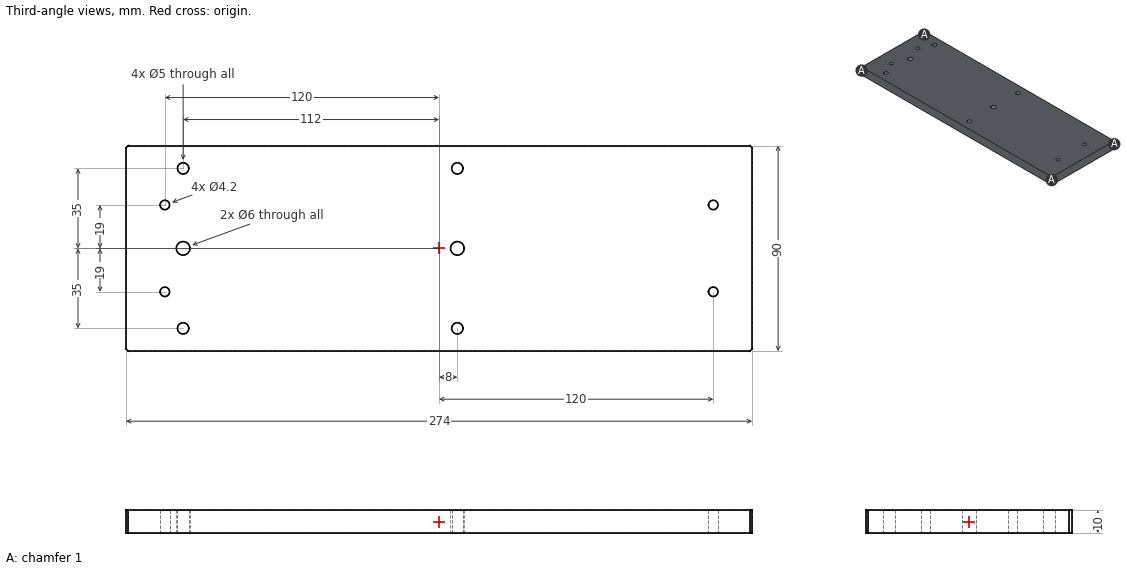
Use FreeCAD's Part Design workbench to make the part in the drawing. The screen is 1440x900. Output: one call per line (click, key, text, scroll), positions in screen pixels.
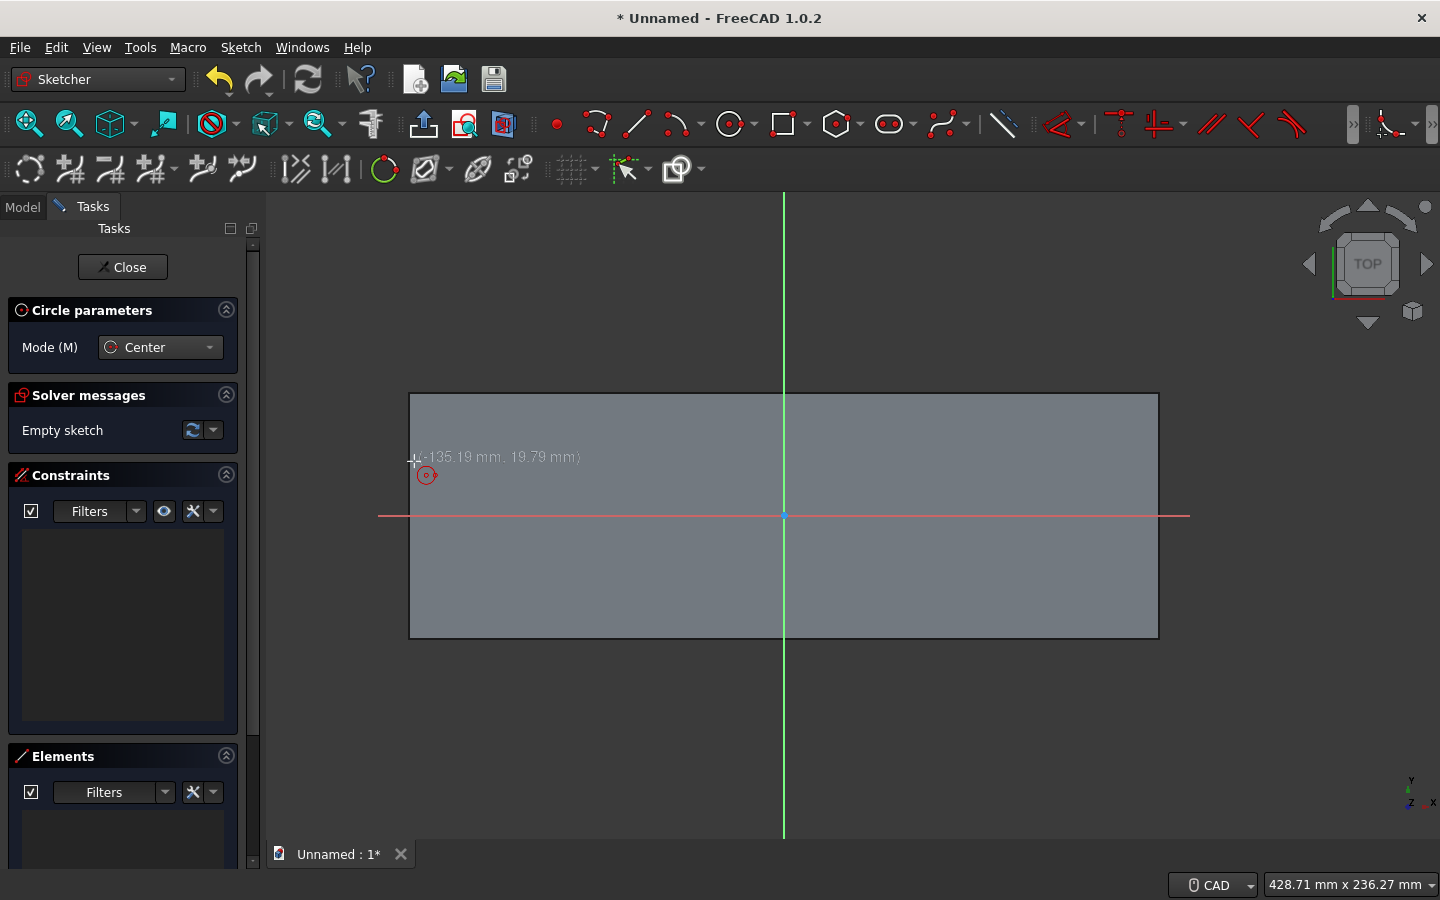
click(456, 464)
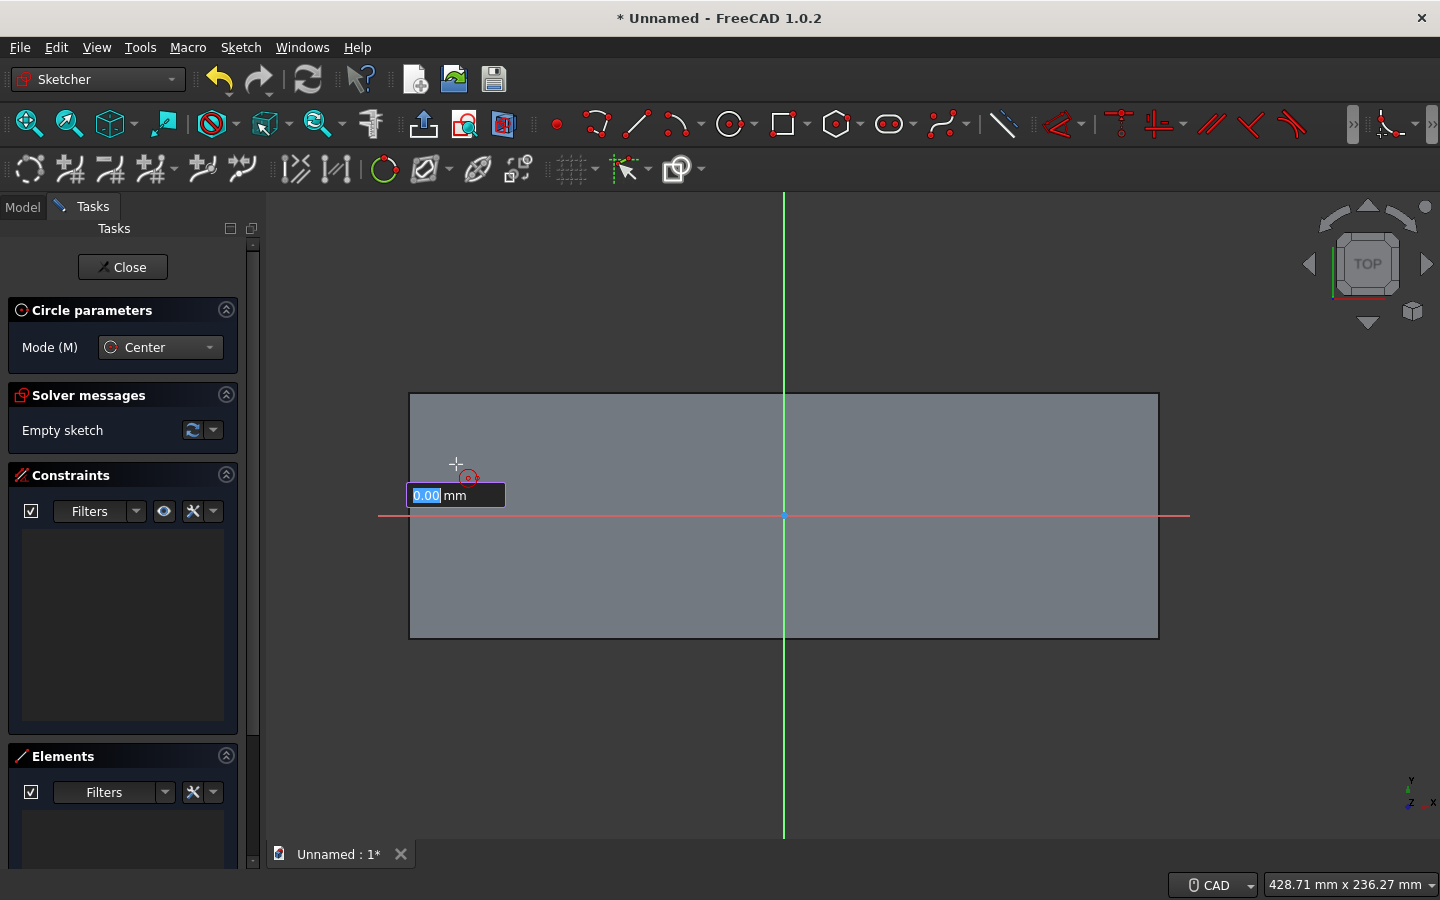
scroll(460, 460, up, 6)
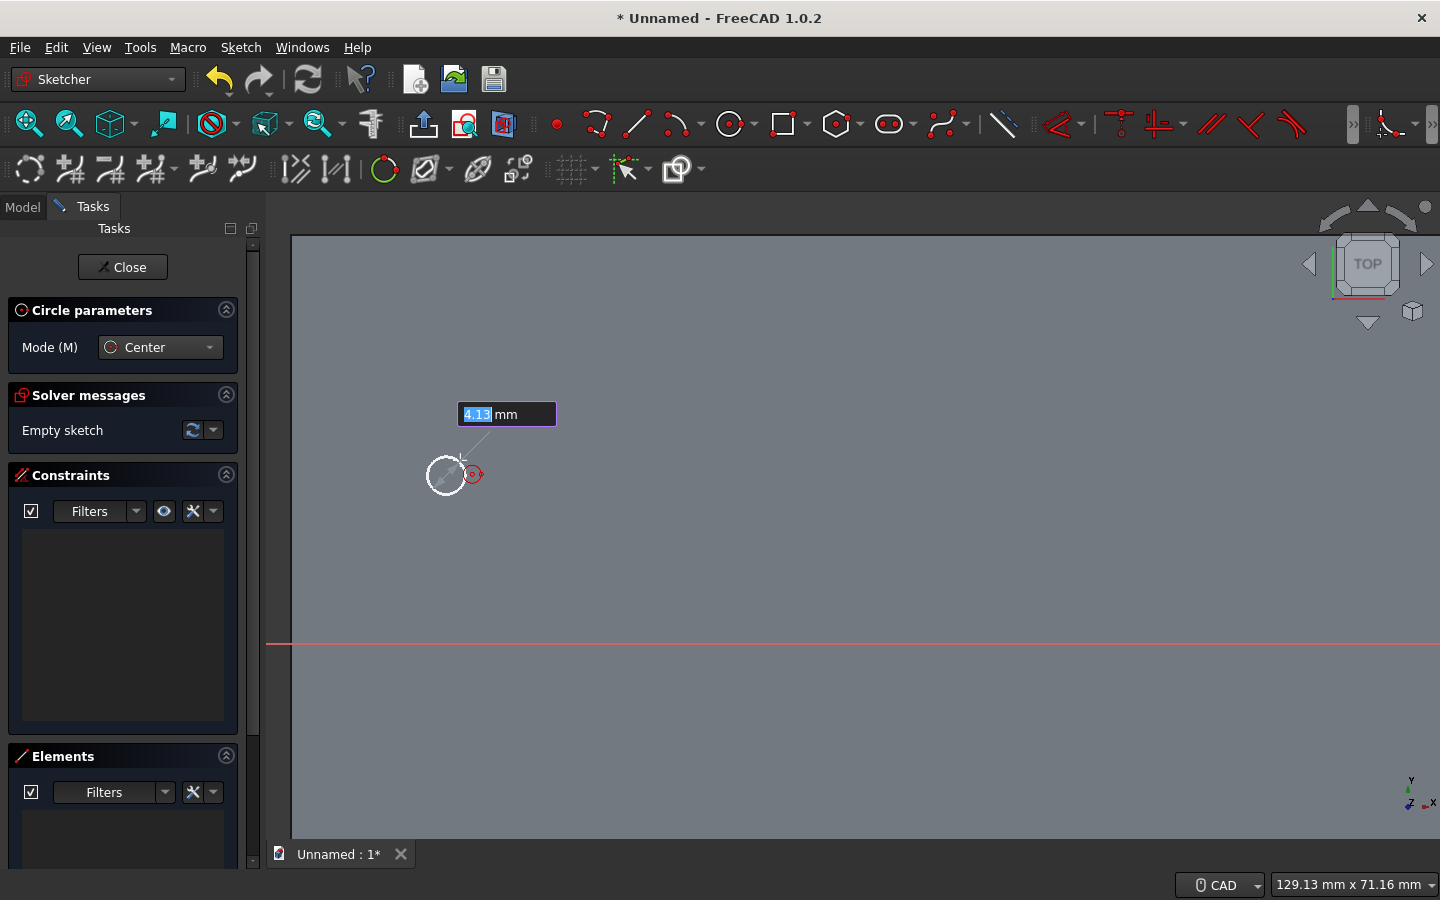
click(459, 458)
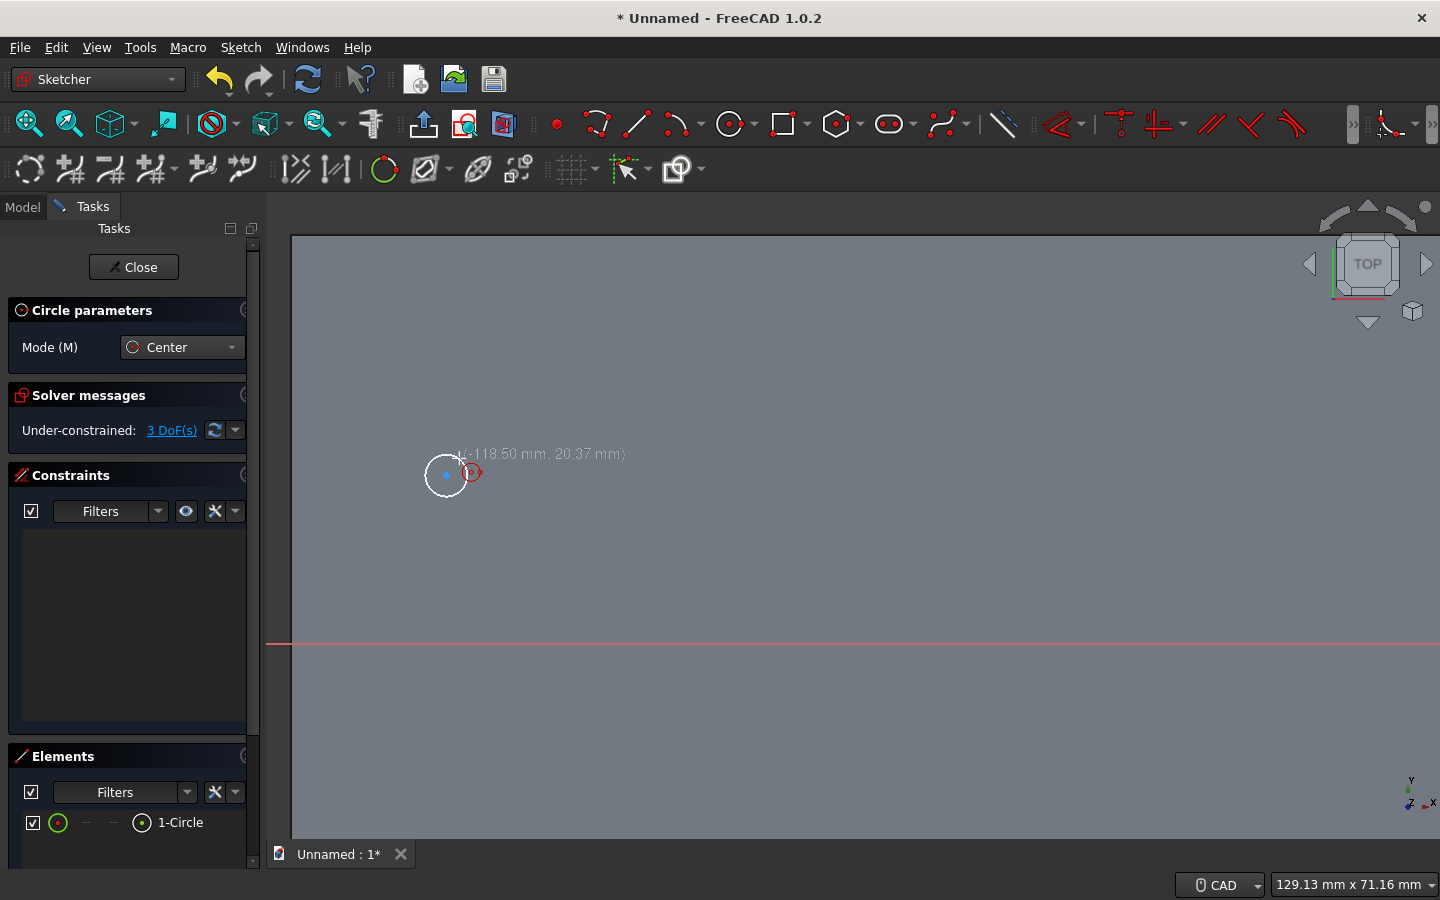
scroll(460, 460, down, 6)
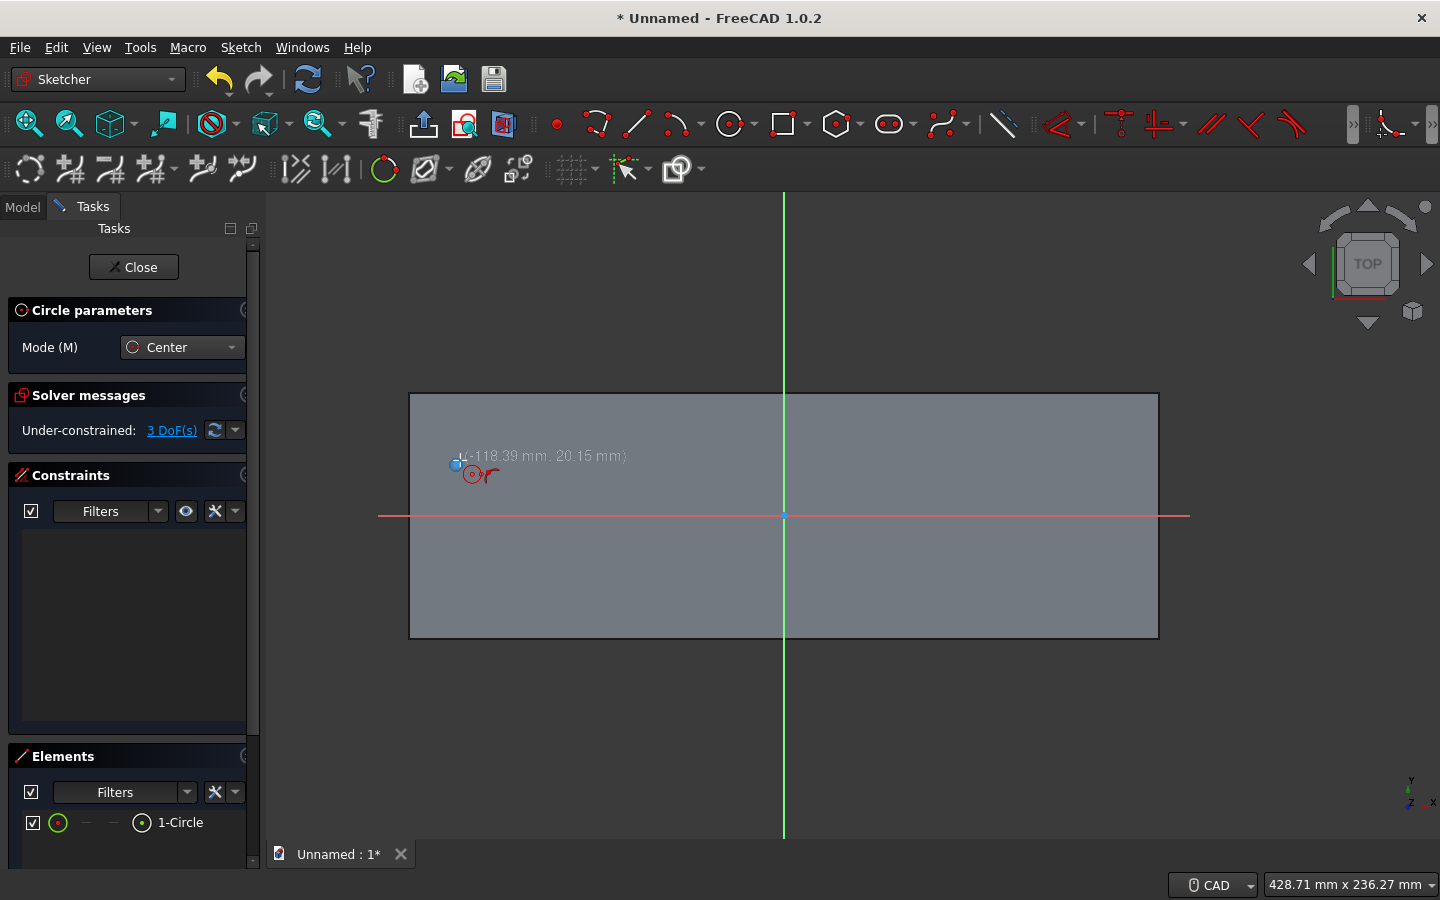
scroll(456, 568, up, 7)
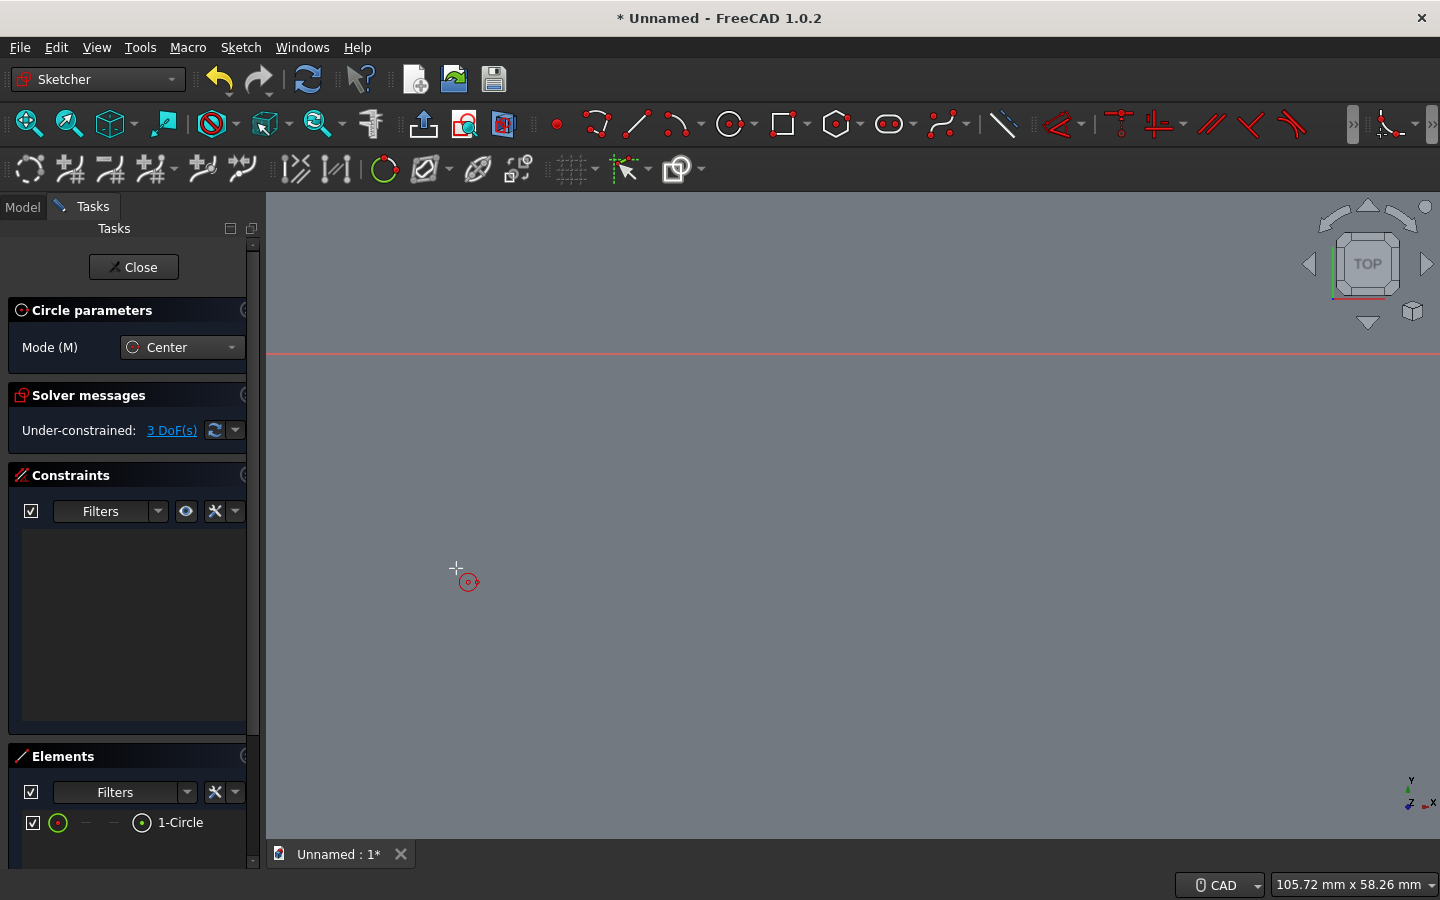
scroll(456, 568, down, 7)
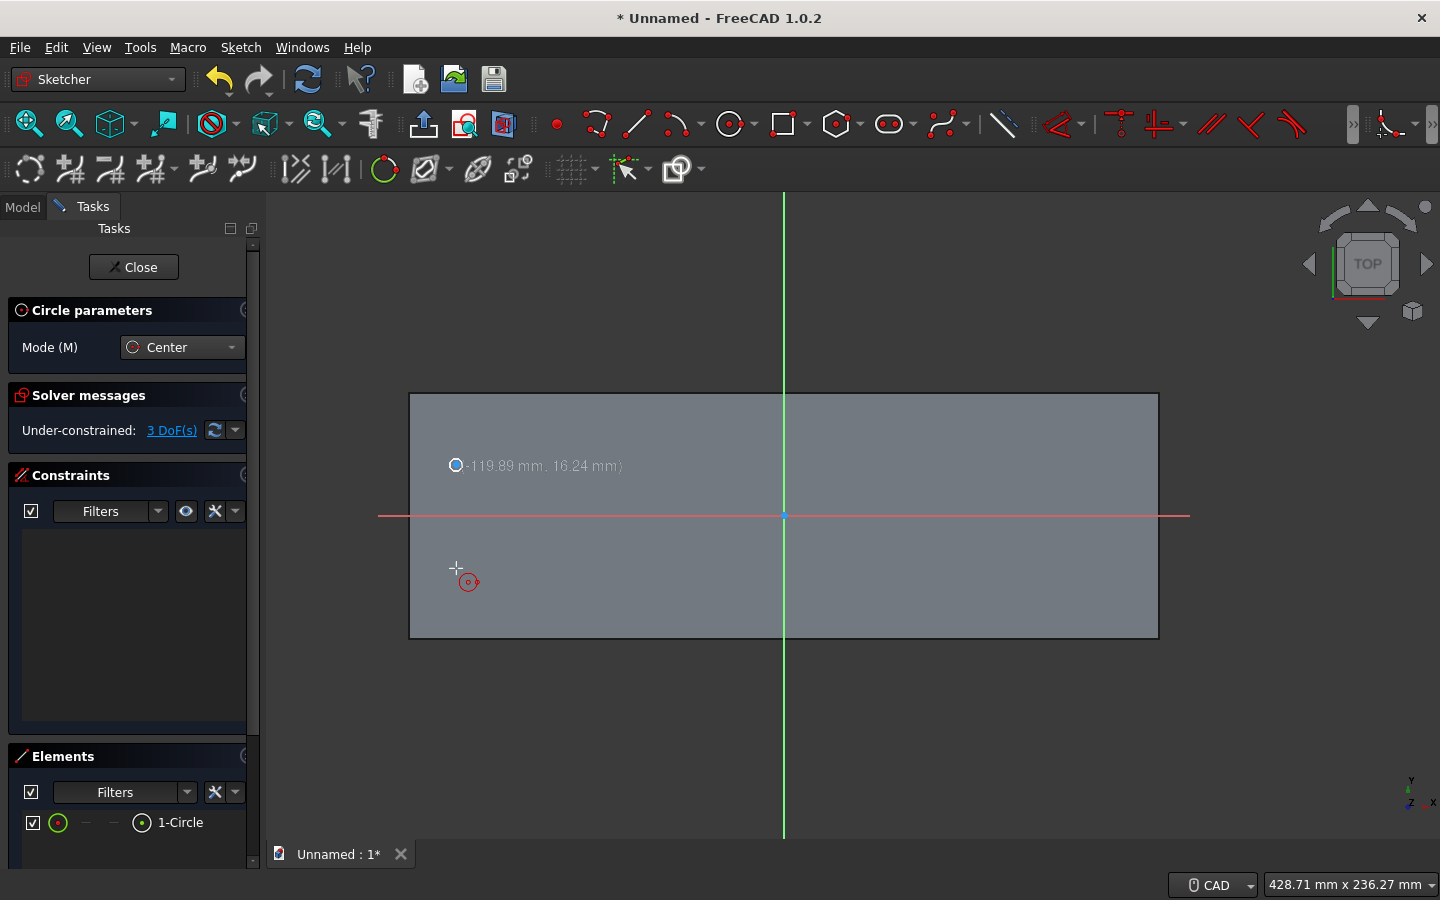
click(456, 568)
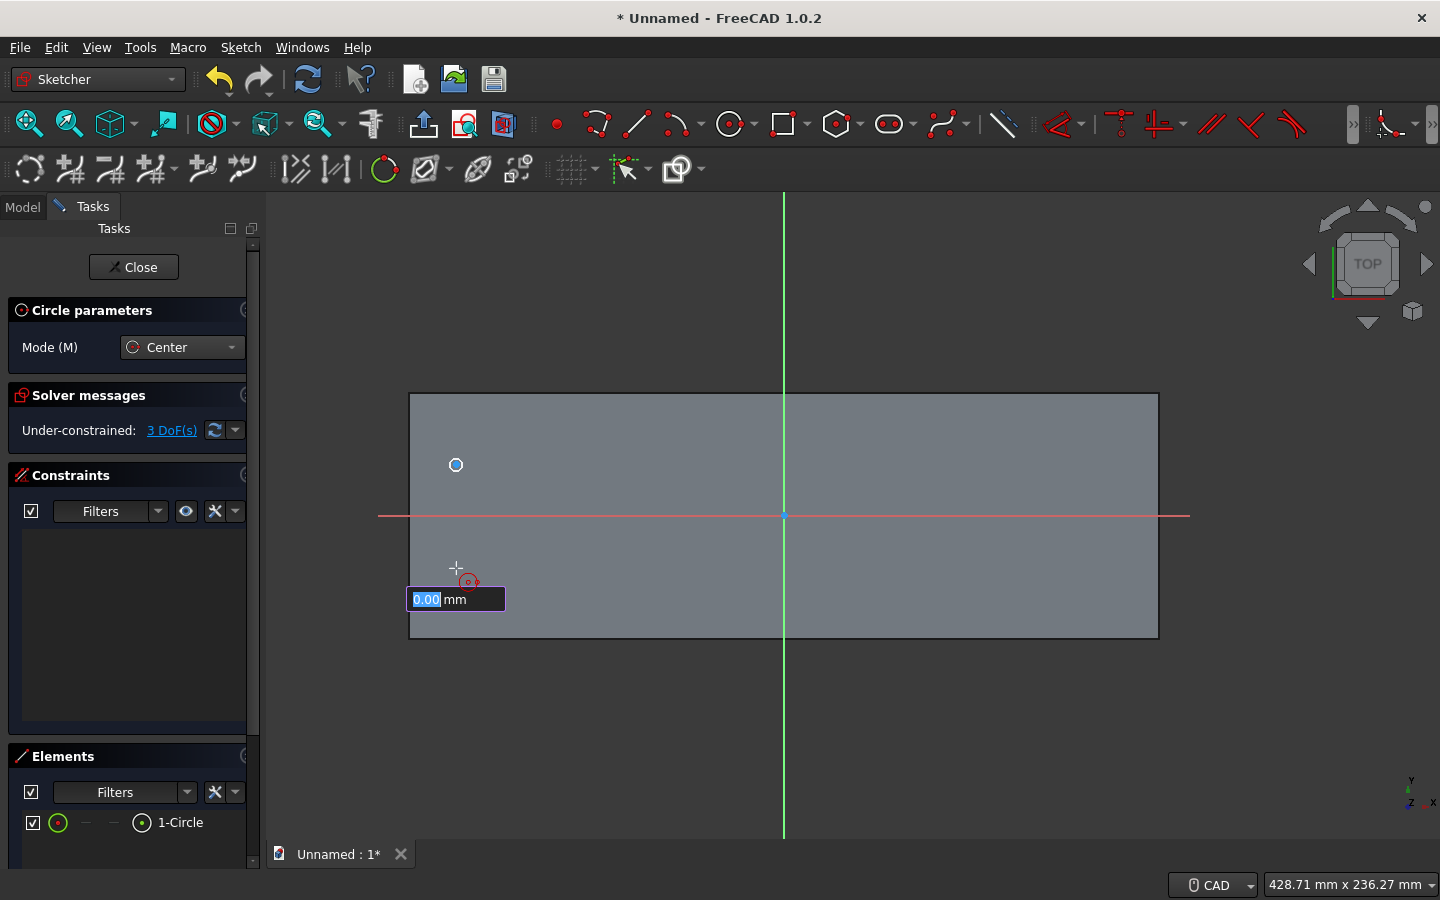
scroll(460, 564, up, 6)